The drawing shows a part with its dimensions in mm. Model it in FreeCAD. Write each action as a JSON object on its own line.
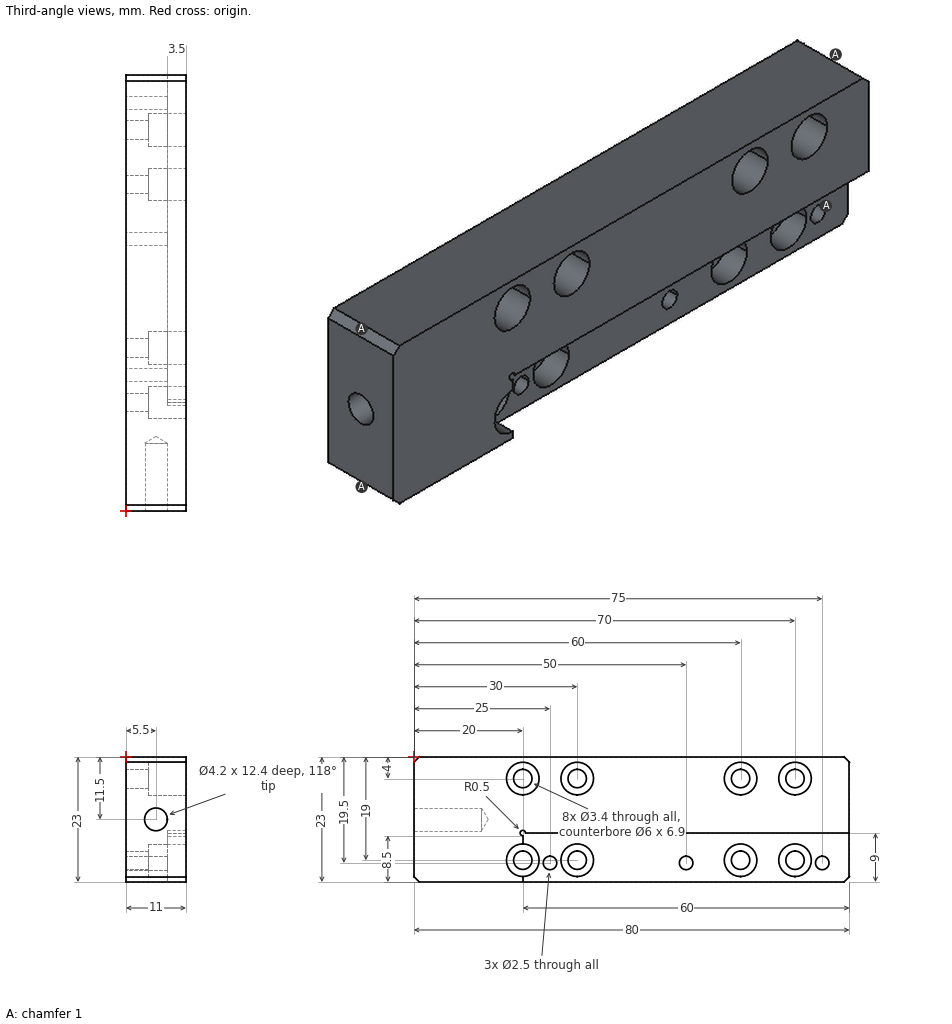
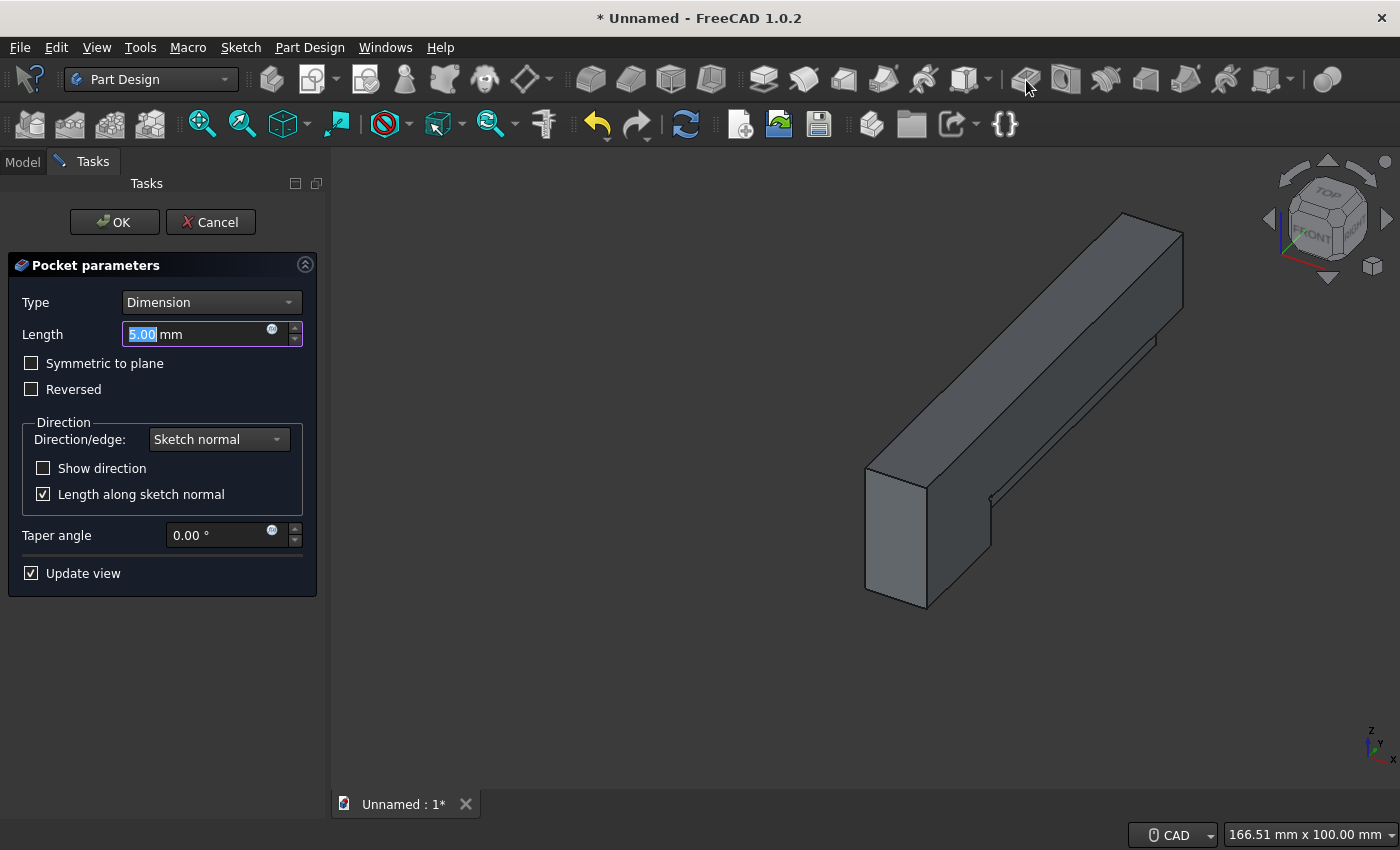
{"action": "type", "text": "3.5"}
{"action": "key", "text": "Tab"}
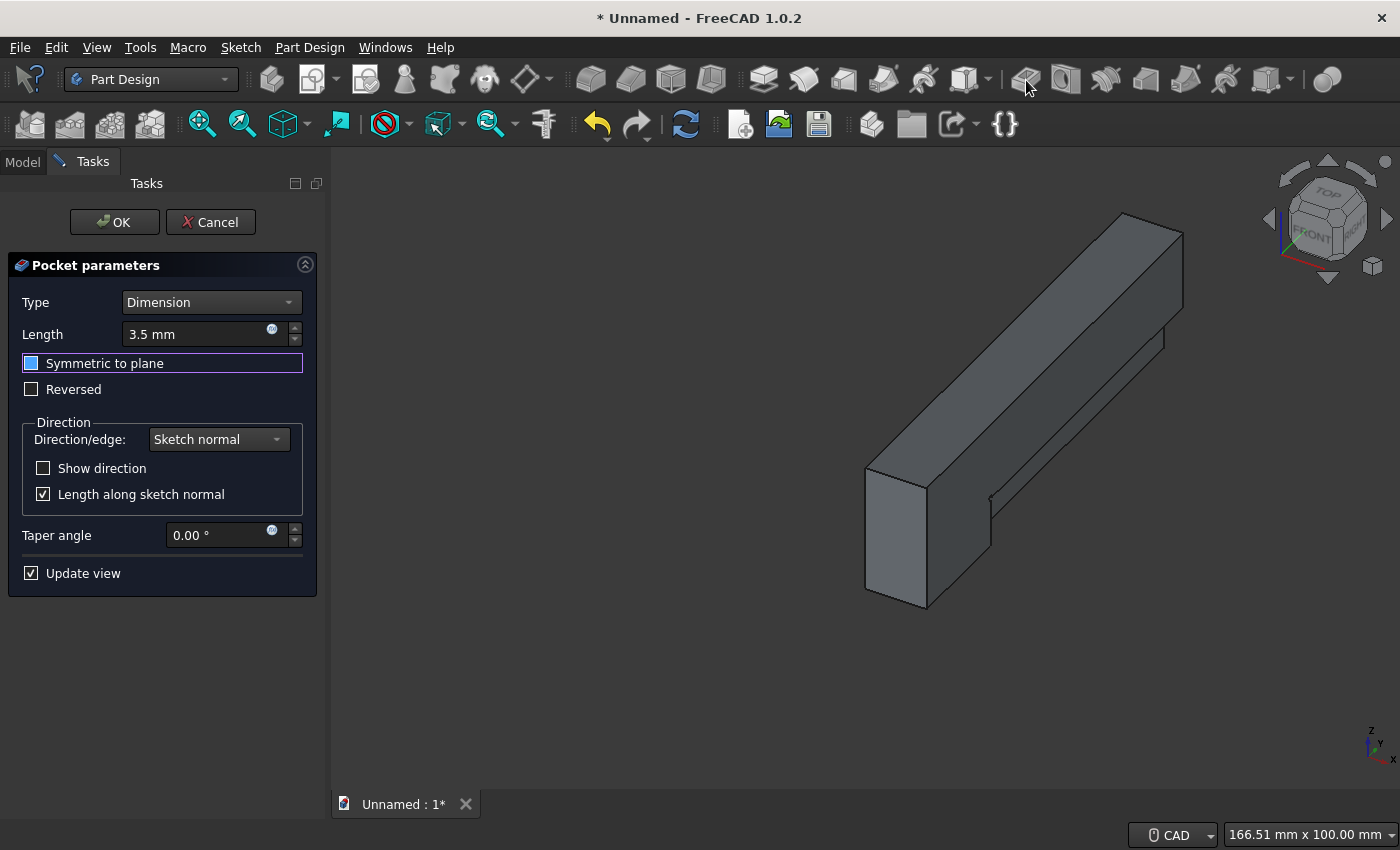
{"action": "left_click", "coordinate": [115, 222]}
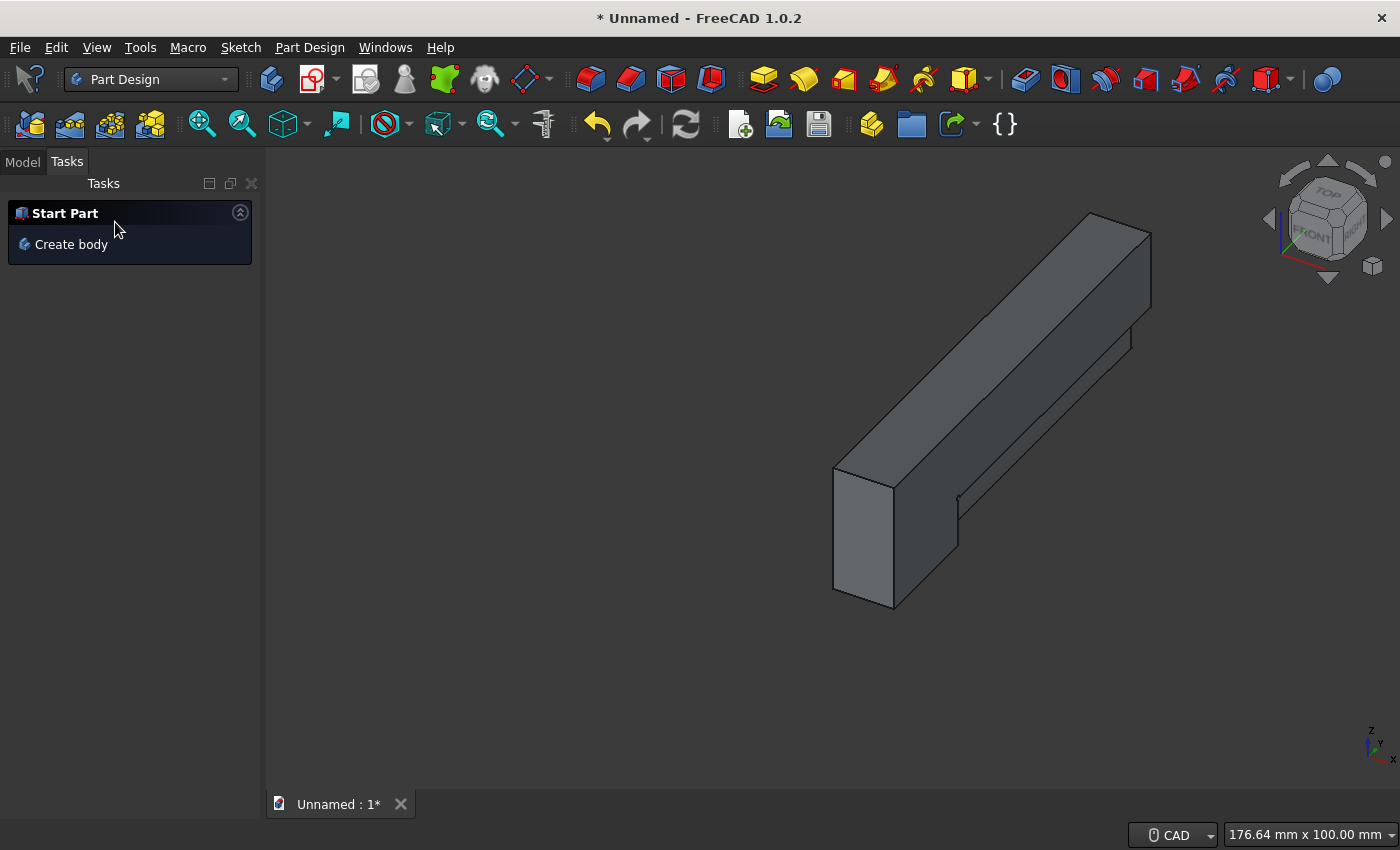
{"action": "left_click", "coordinate": [949, 476]}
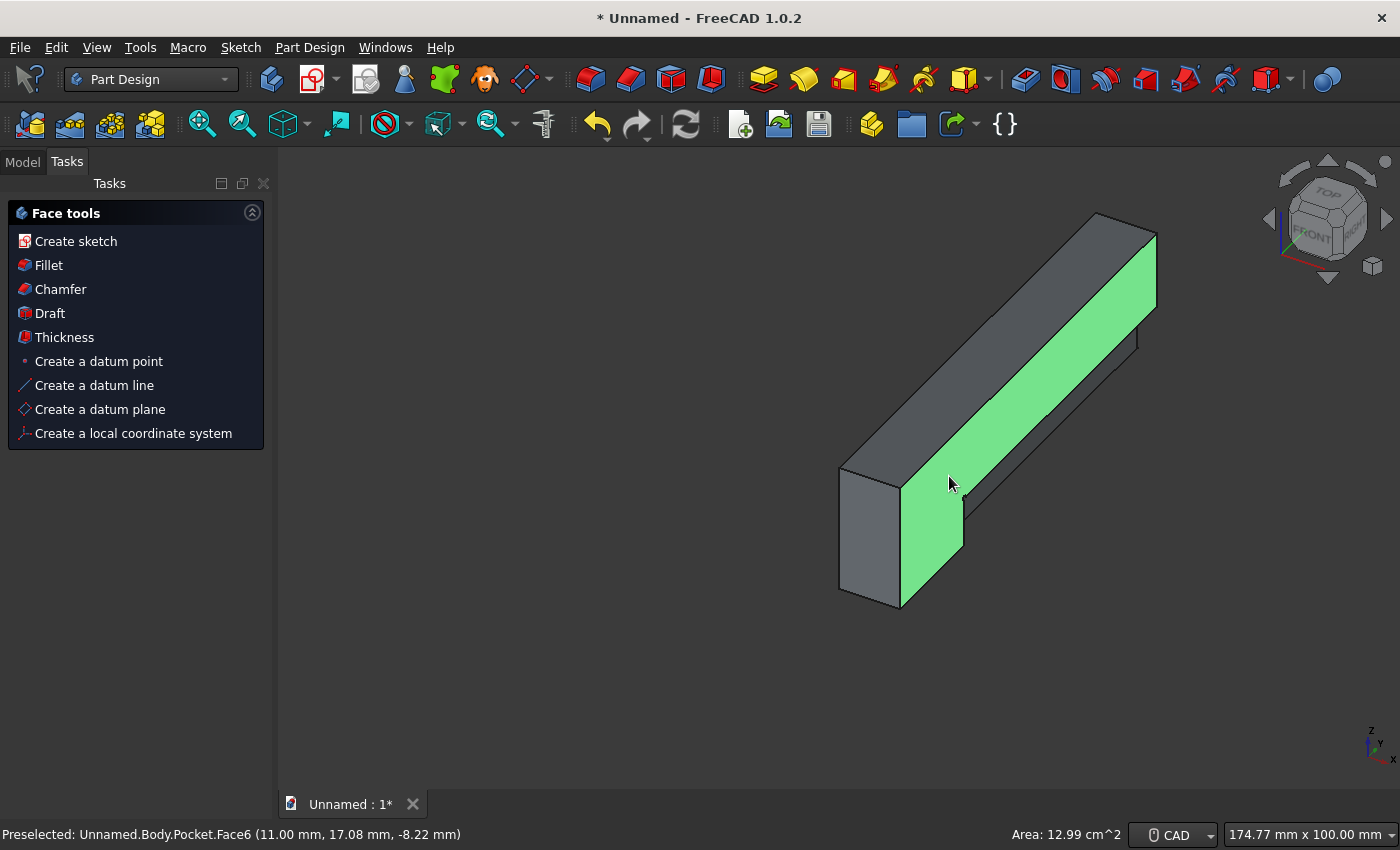
{"action": "left_click", "coordinate": [312, 80]}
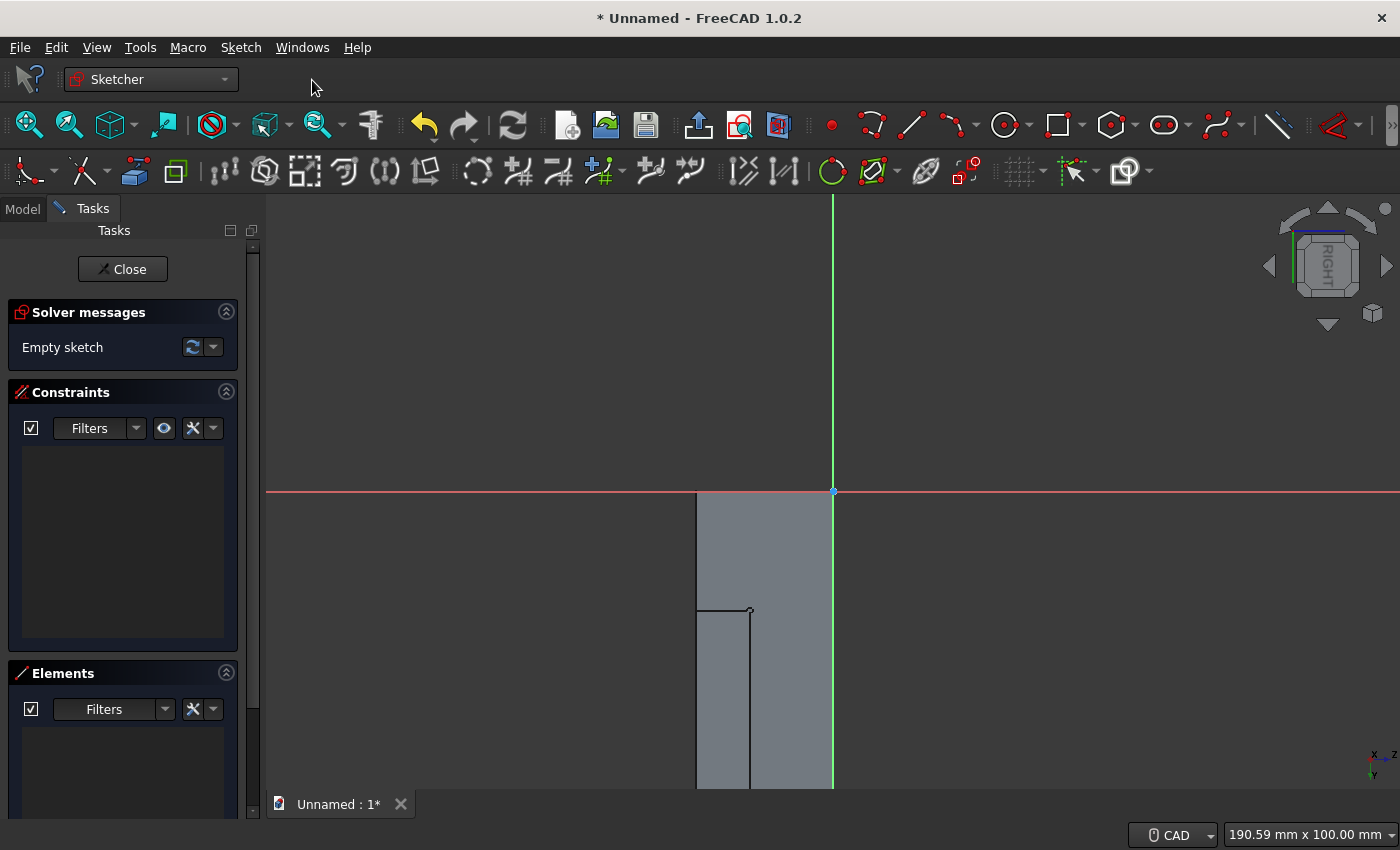
{"action": "scroll", "coordinate": [750, 222], "scroll_direction": "down", "scroll_amount": 2}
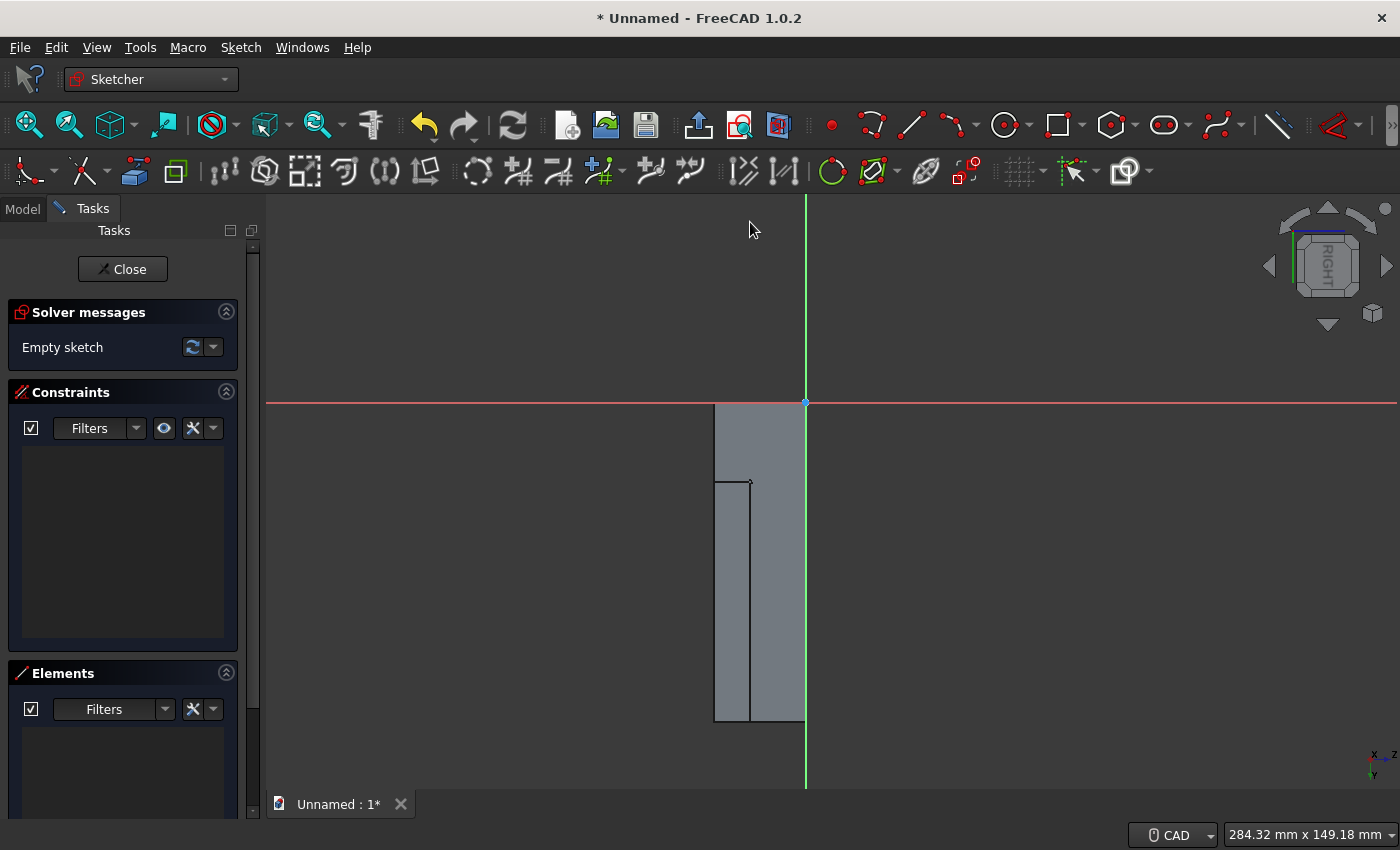
{"action": "left_click", "coordinate": [1006, 126]}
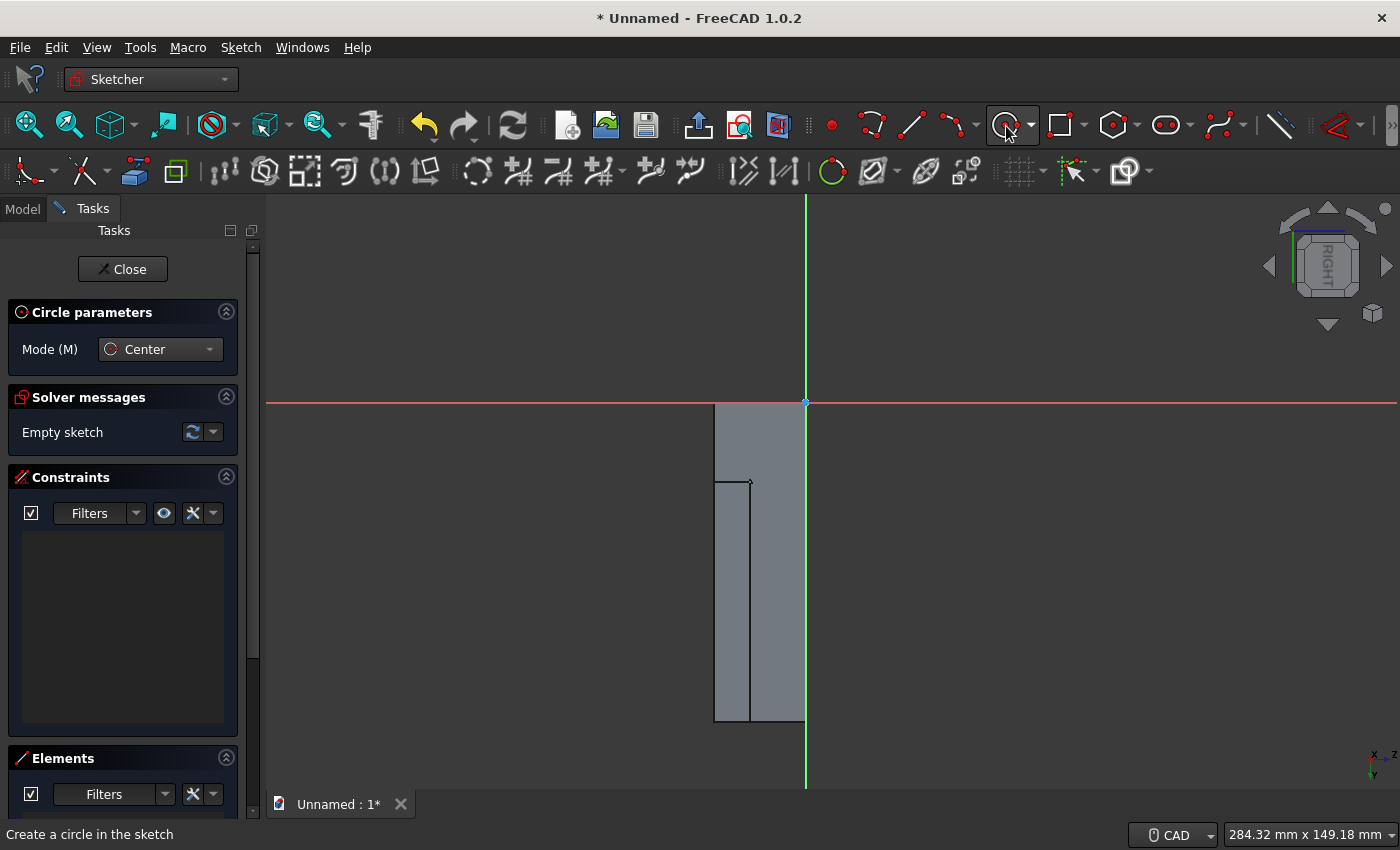
{"action": "scroll", "coordinate": [790, 482], "scroll_direction": "up", "scroll_amount": 7}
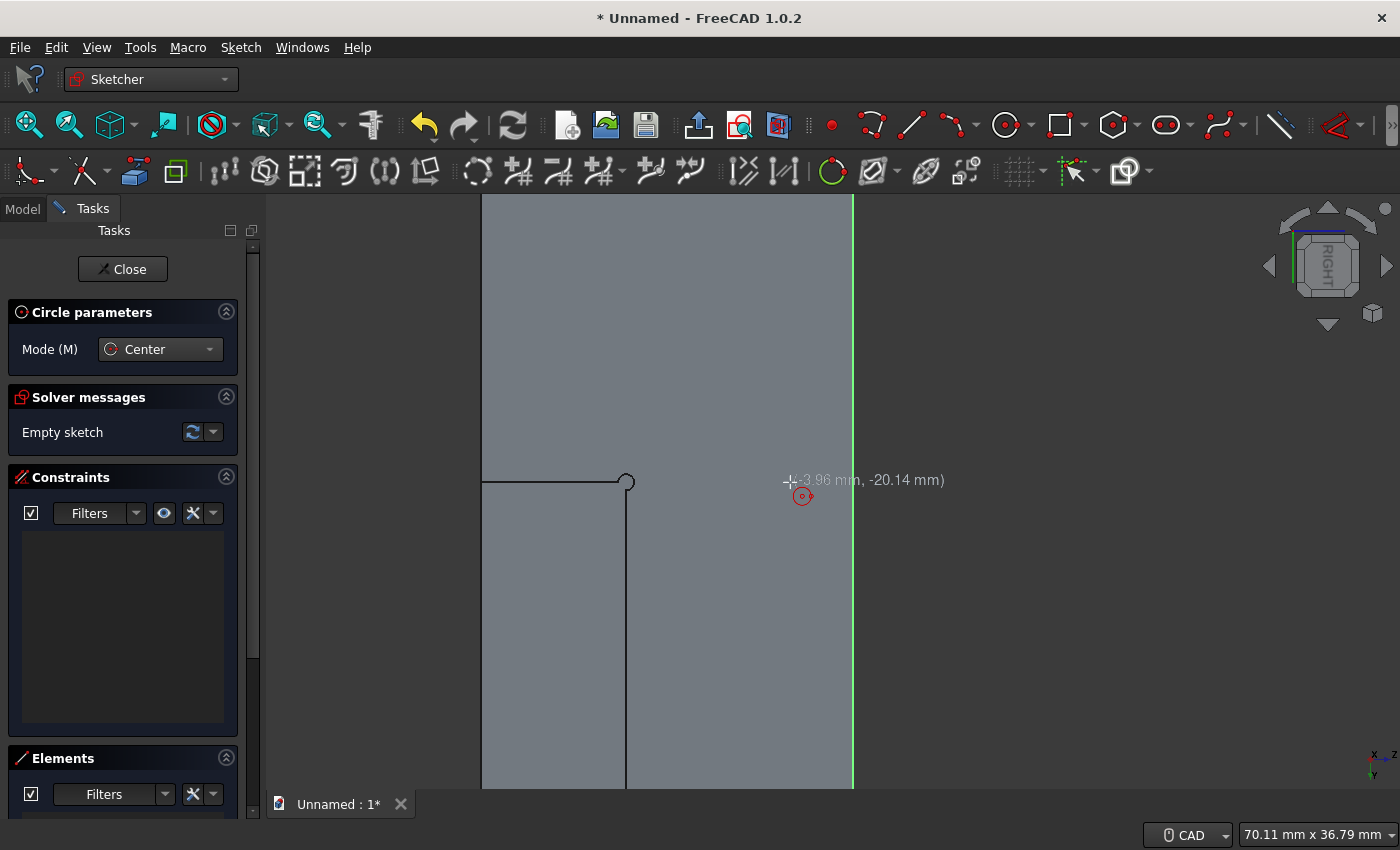
{"action": "scroll", "coordinate": [799, 385], "scroll_direction": "down", "scroll_amount": 6}